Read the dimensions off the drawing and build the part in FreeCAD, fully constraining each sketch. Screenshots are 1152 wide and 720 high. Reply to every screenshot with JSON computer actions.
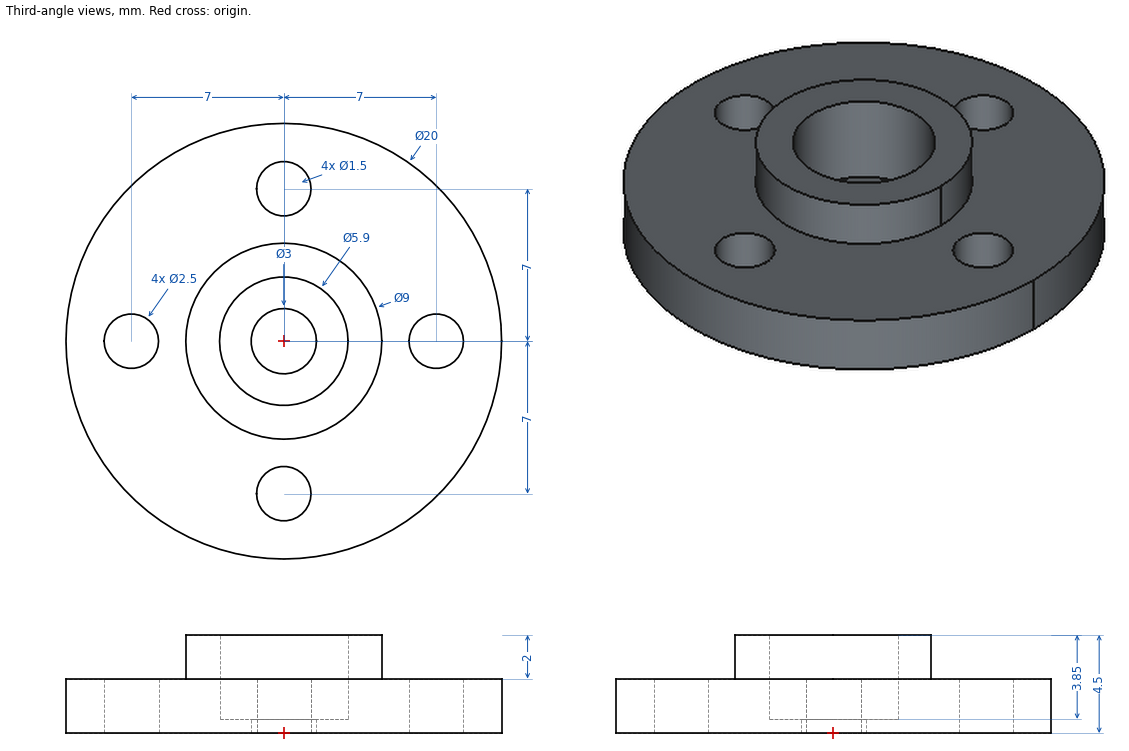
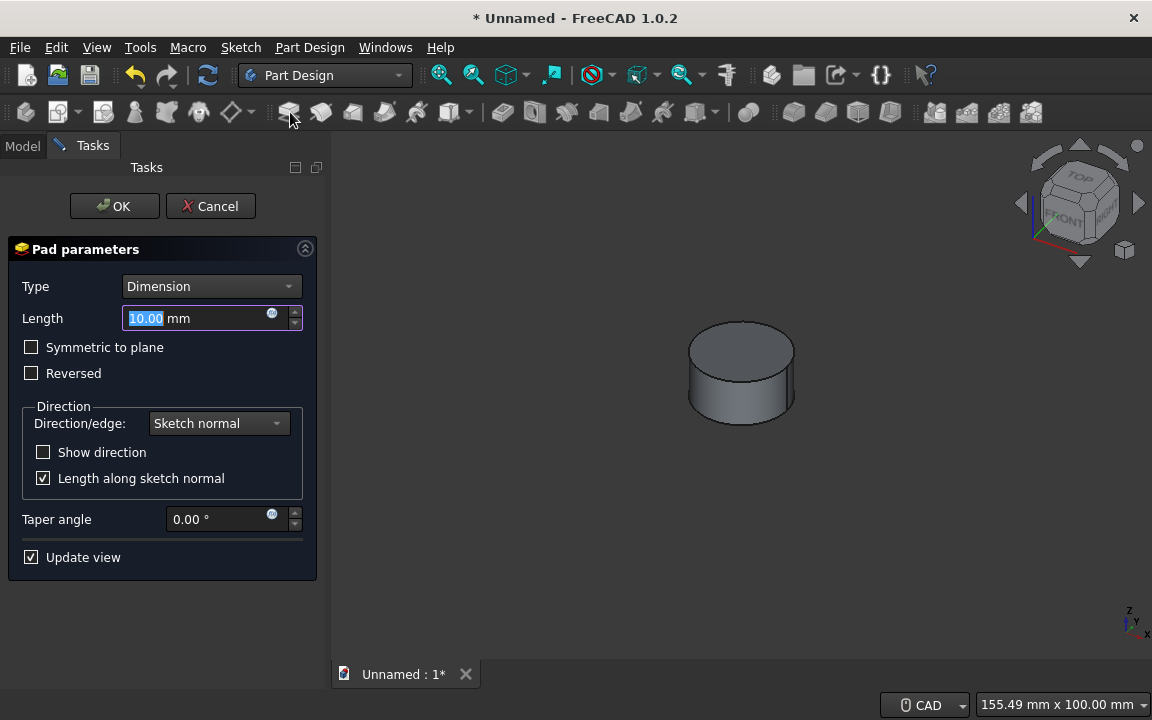
{"action": "type", "text": "4.5"}
{"action": "key", "text": "Tab"}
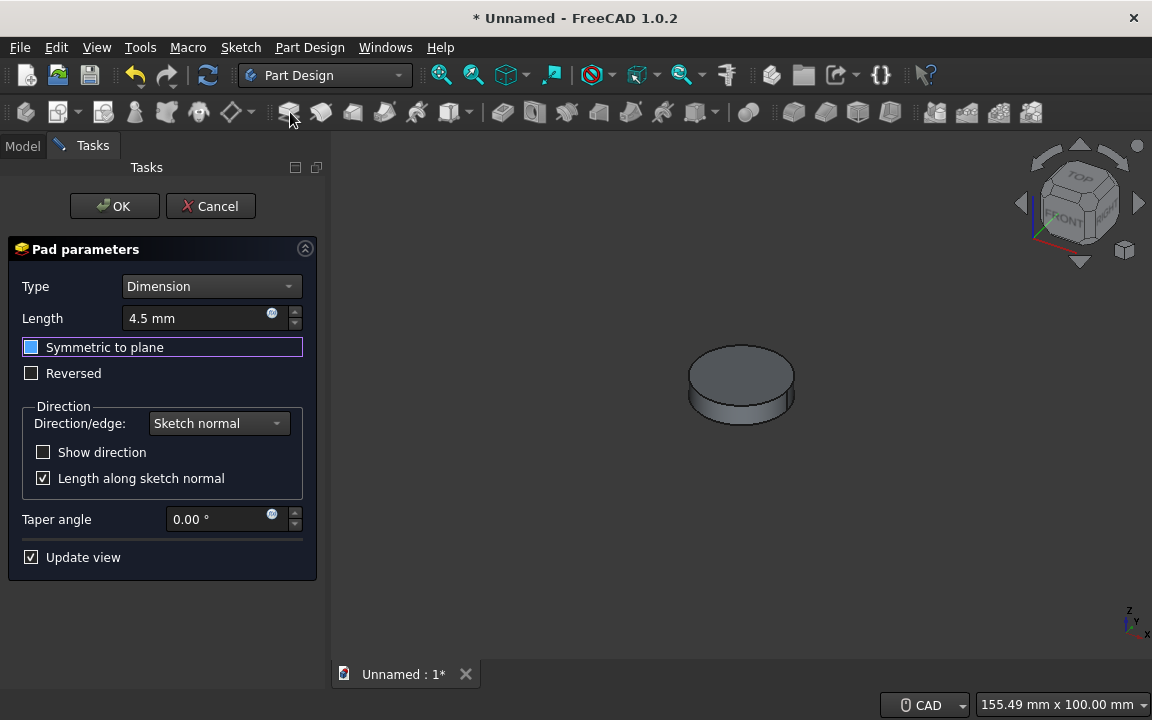
{"action": "left_click", "coordinate": [115, 206]}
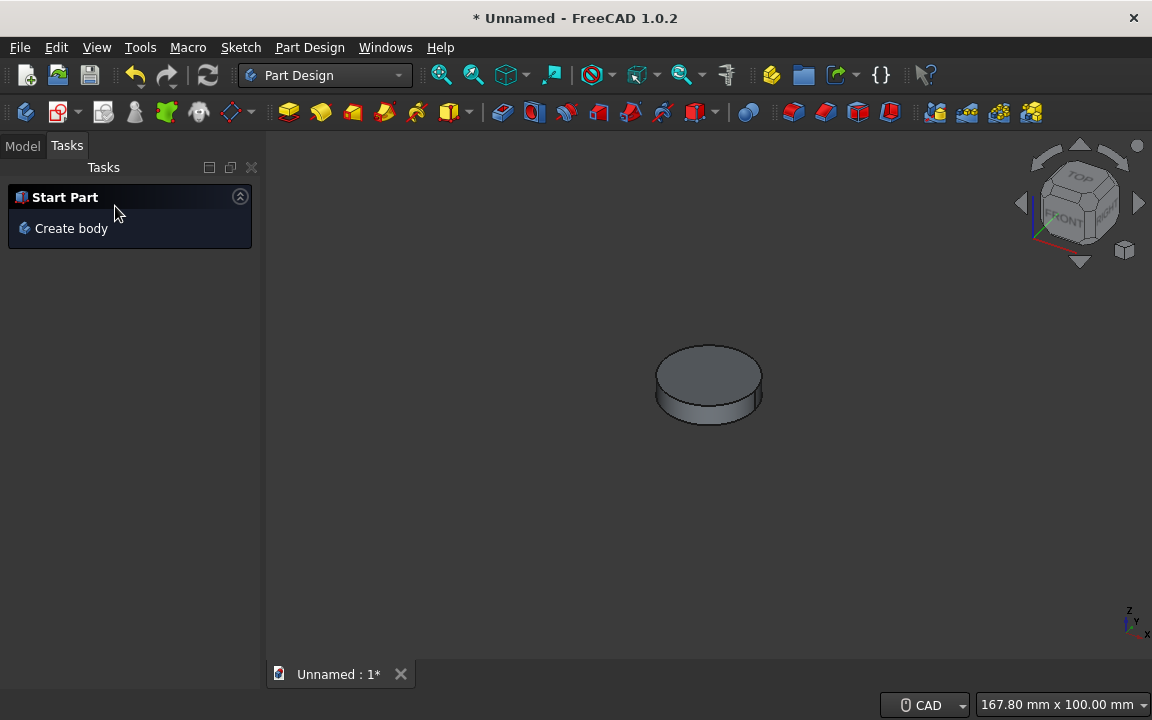
{"action": "key", "text": "v f"}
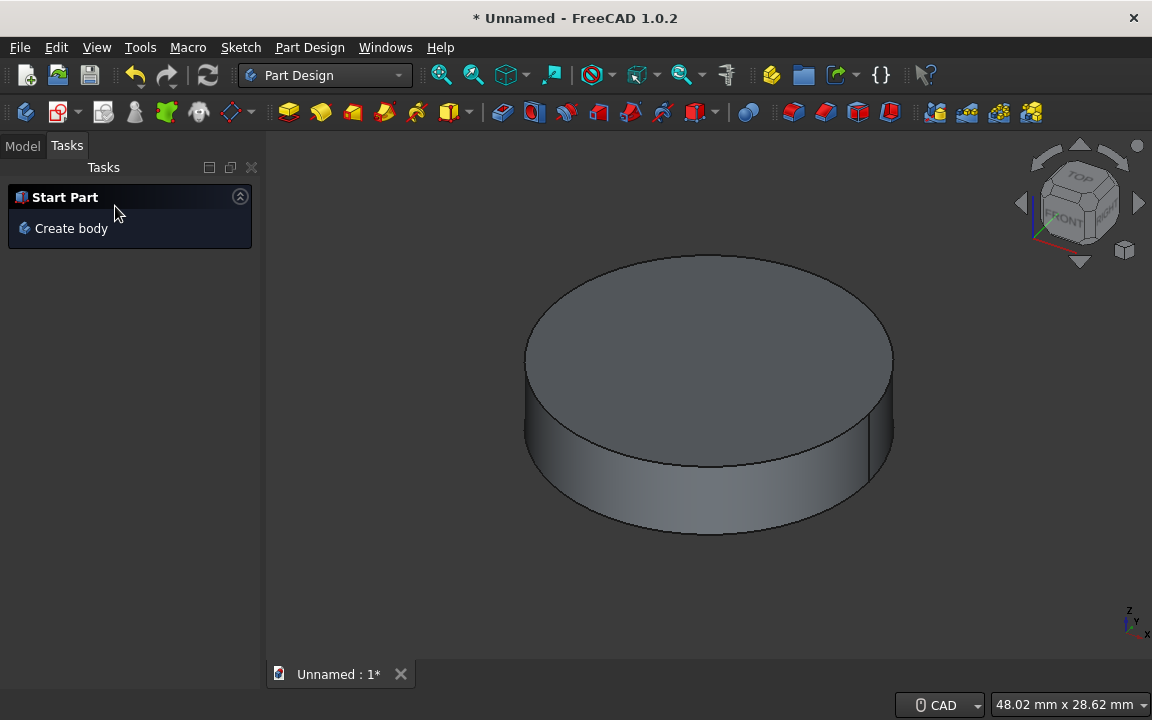
{"action": "left_click", "coordinate": [23, 145]}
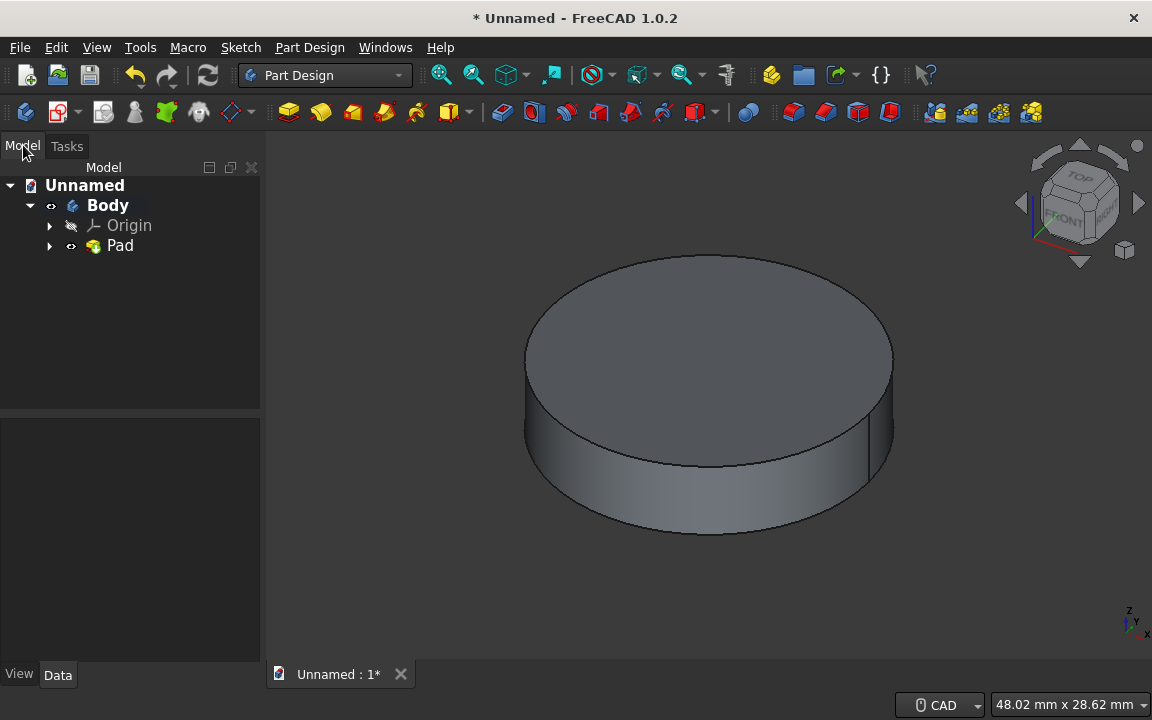
{"action": "left_click", "coordinate": [50, 226]}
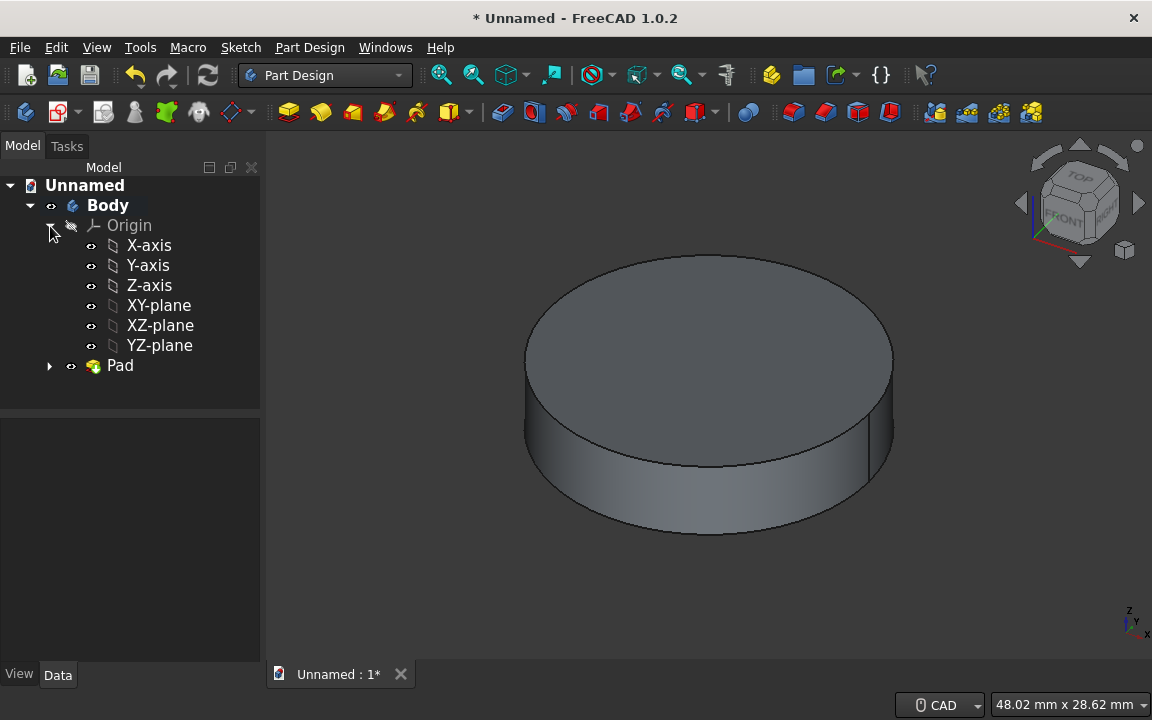
{"action": "left_click", "coordinate": [136, 306]}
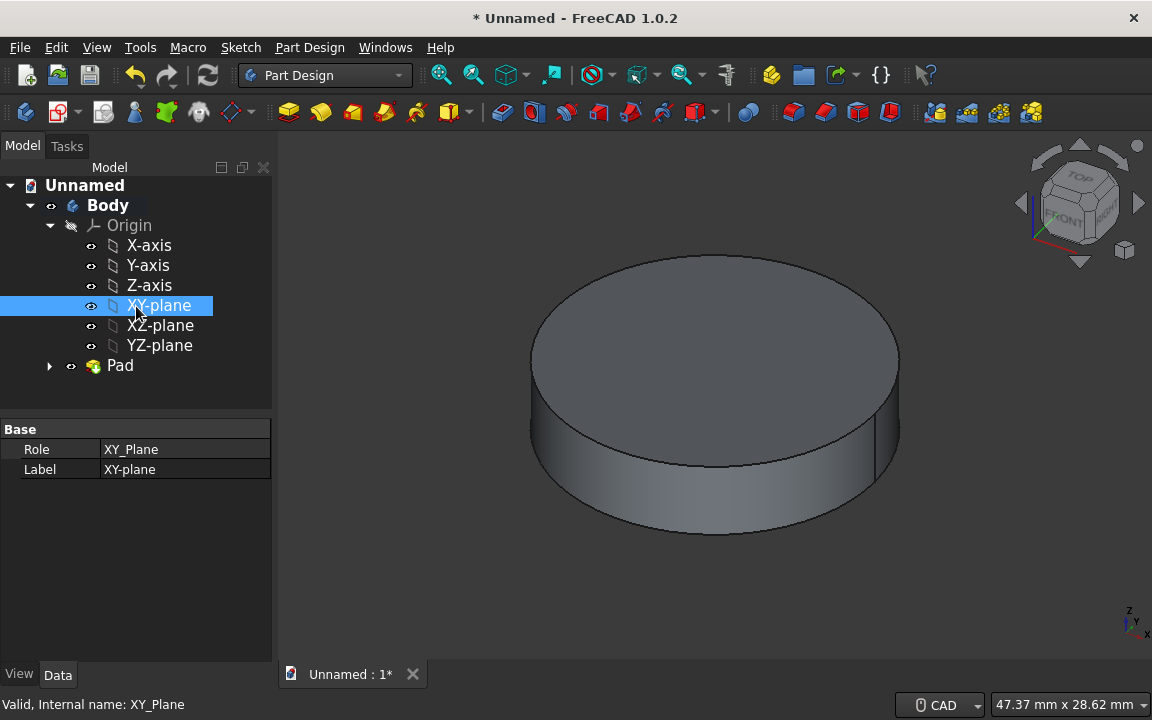
{"action": "left_click", "coordinate": [232, 112]}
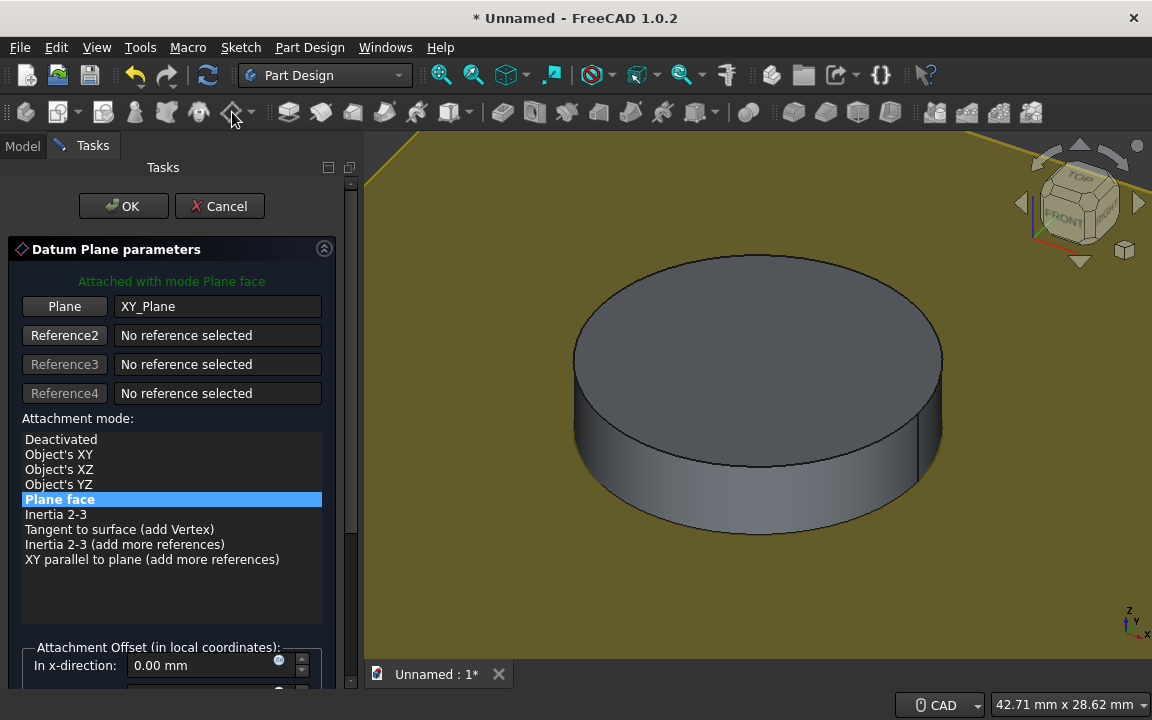
{"action": "scroll", "coordinate": [351, 432], "scroll_direction": "down", "scroll_amount": 2}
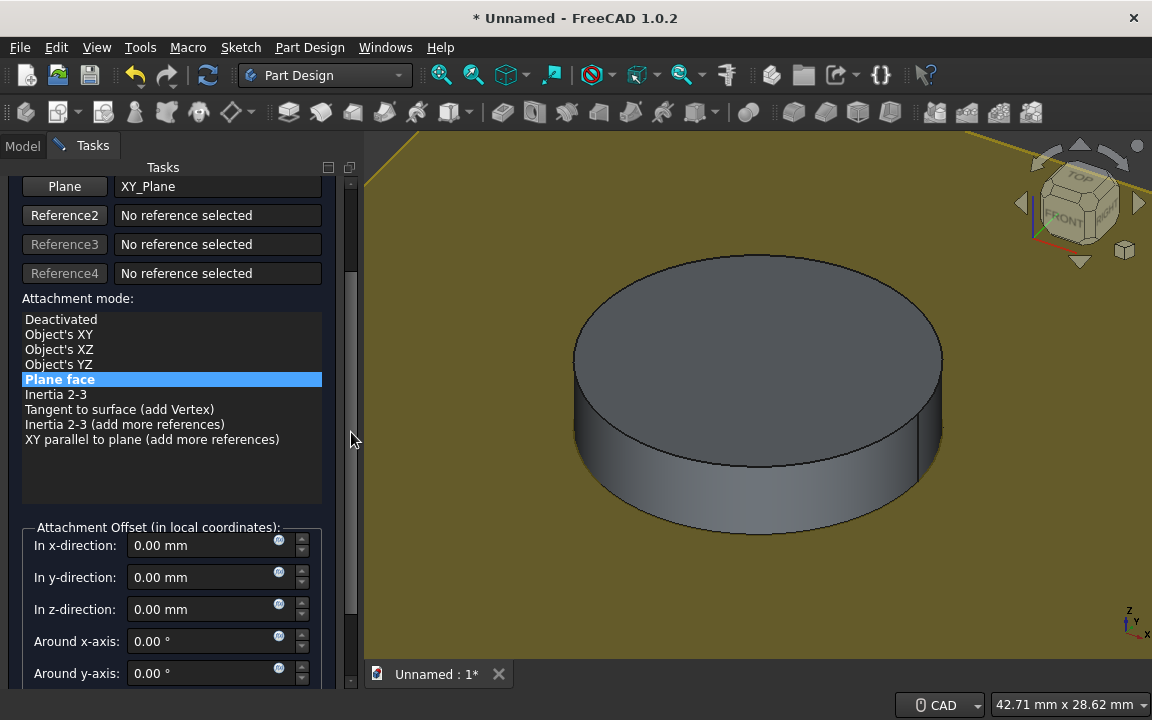
{"action": "triple_click", "coordinate": [210, 609]}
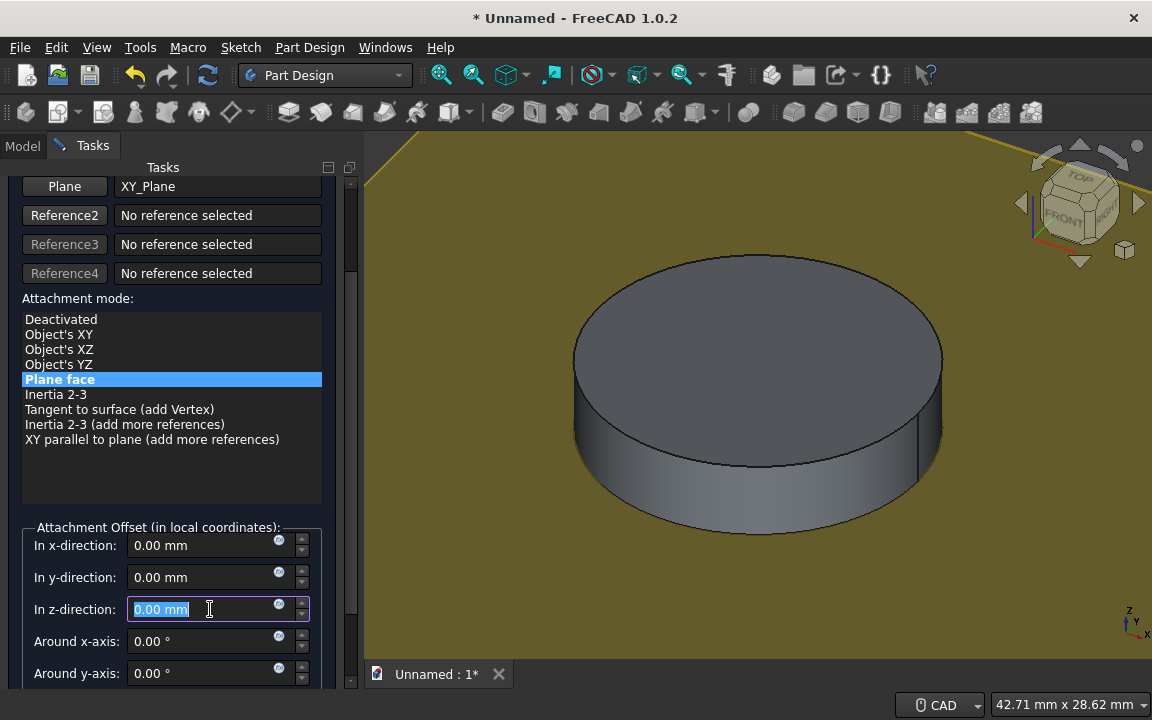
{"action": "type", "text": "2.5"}
{"action": "key", "text": "Tab"}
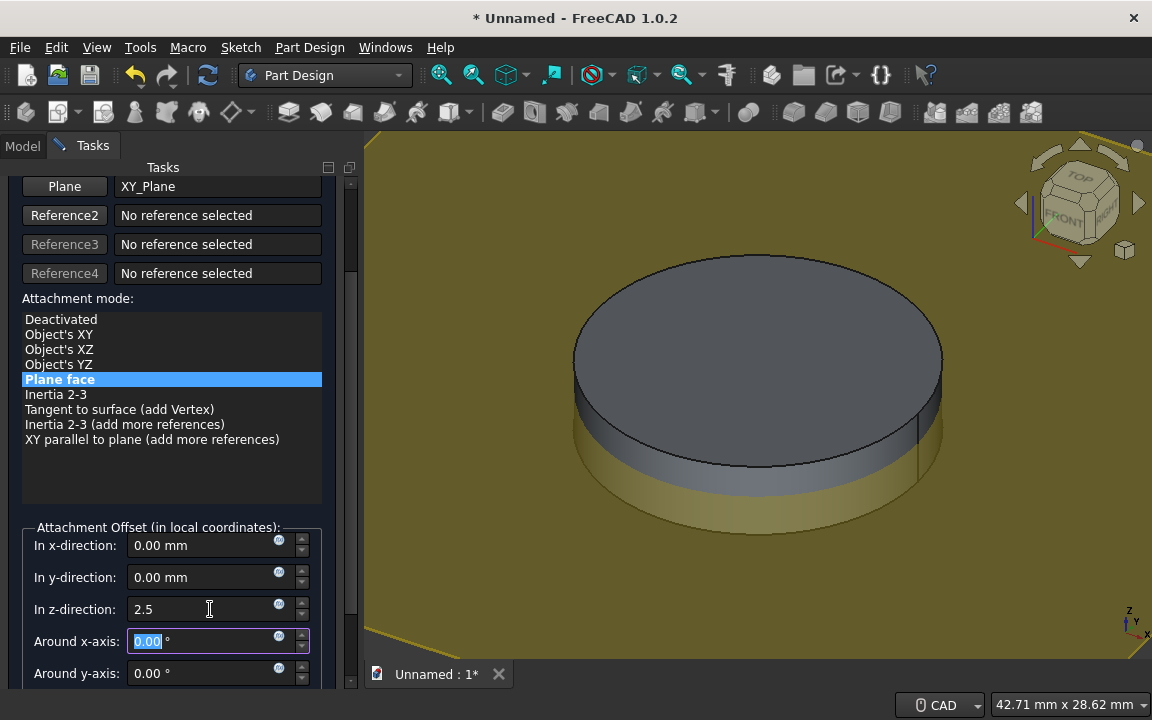
{"action": "scroll", "coordinate": [351, 432], "scroll_direction": "up", "scroll_amount": 3}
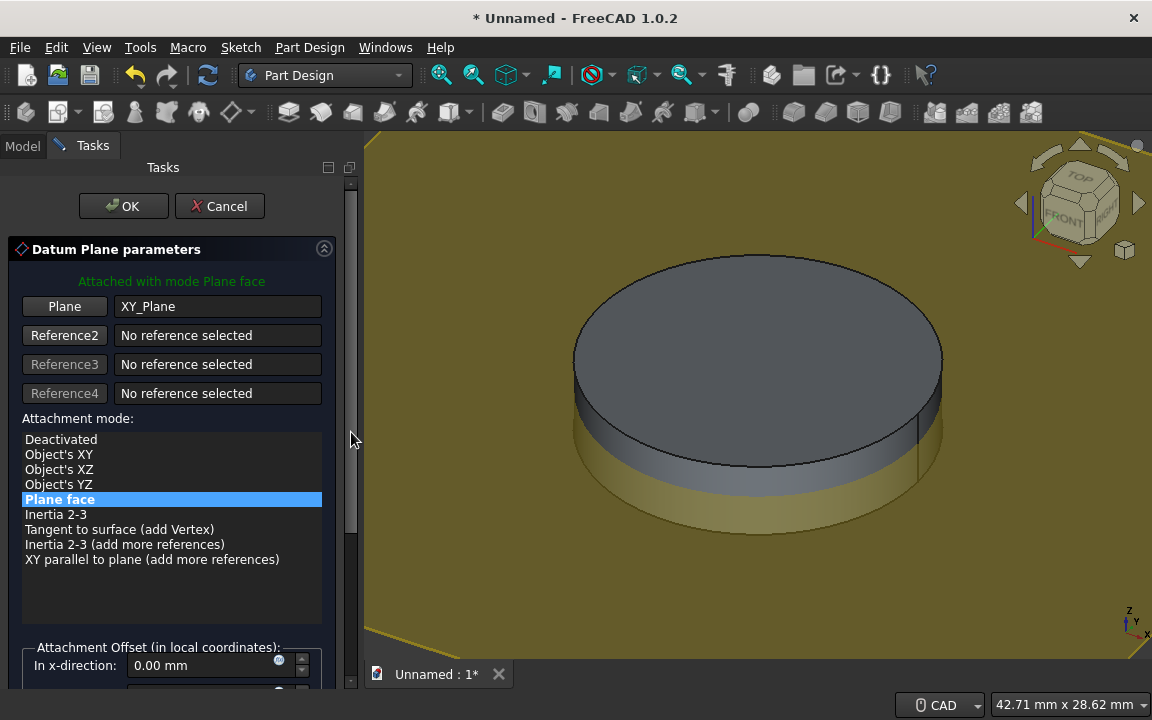
{"action": "left_click", "coordinate": [124, 206]}